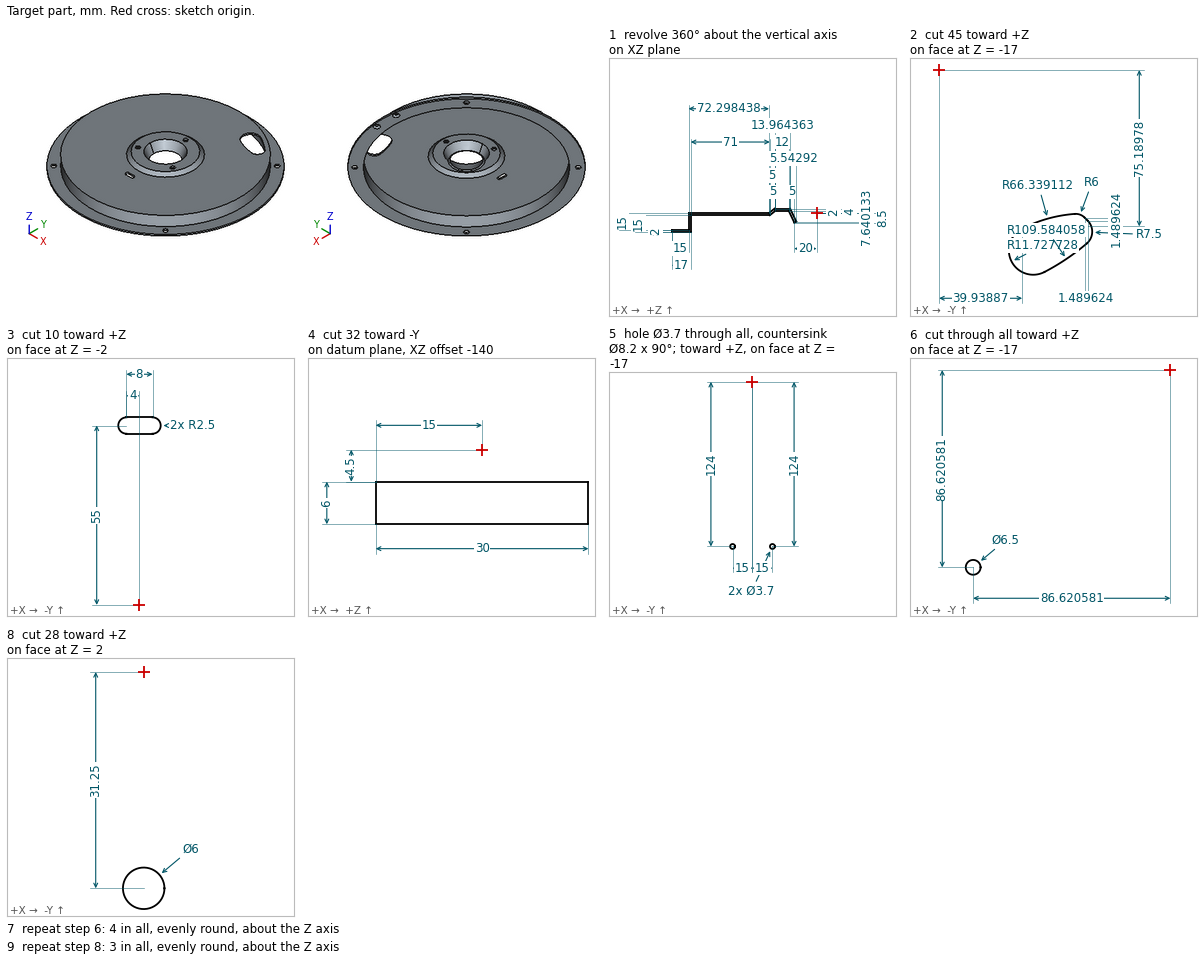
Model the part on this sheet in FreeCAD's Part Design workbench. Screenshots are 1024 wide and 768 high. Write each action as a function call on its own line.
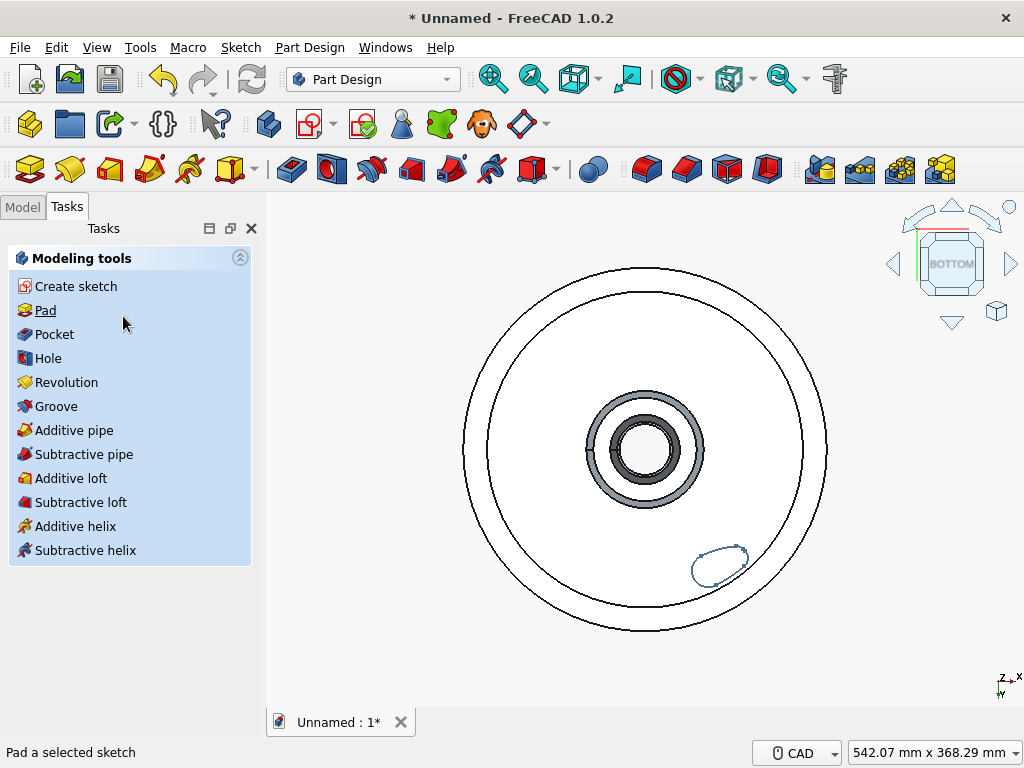
click(292, 170)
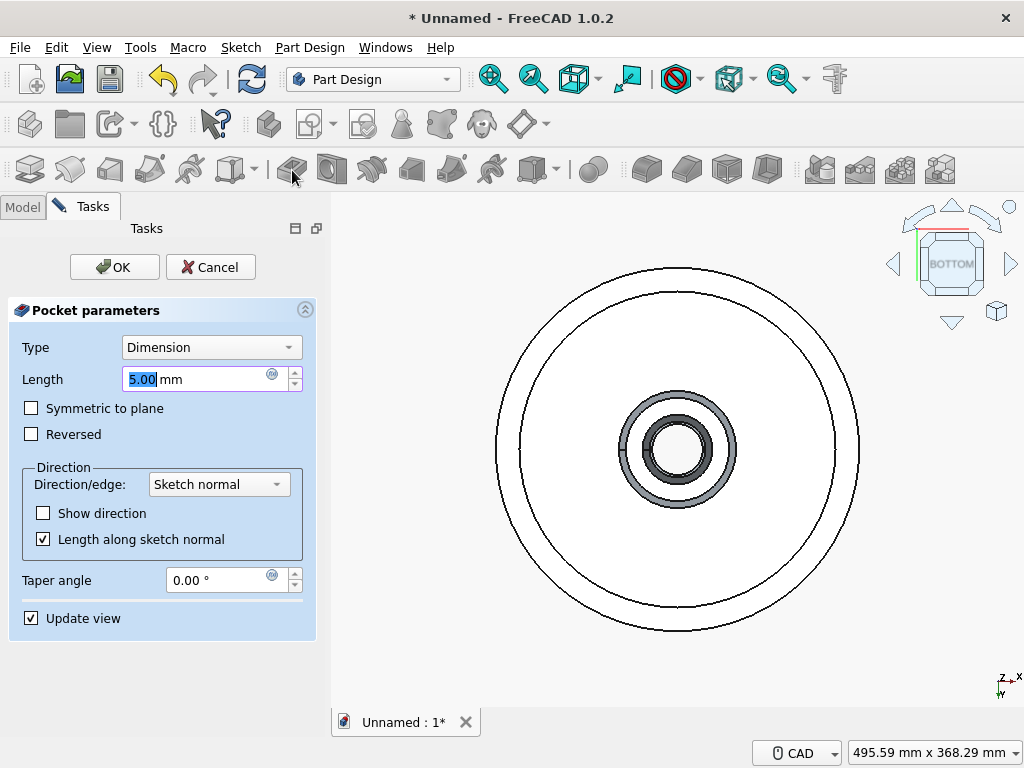
text(45)
key(Tab)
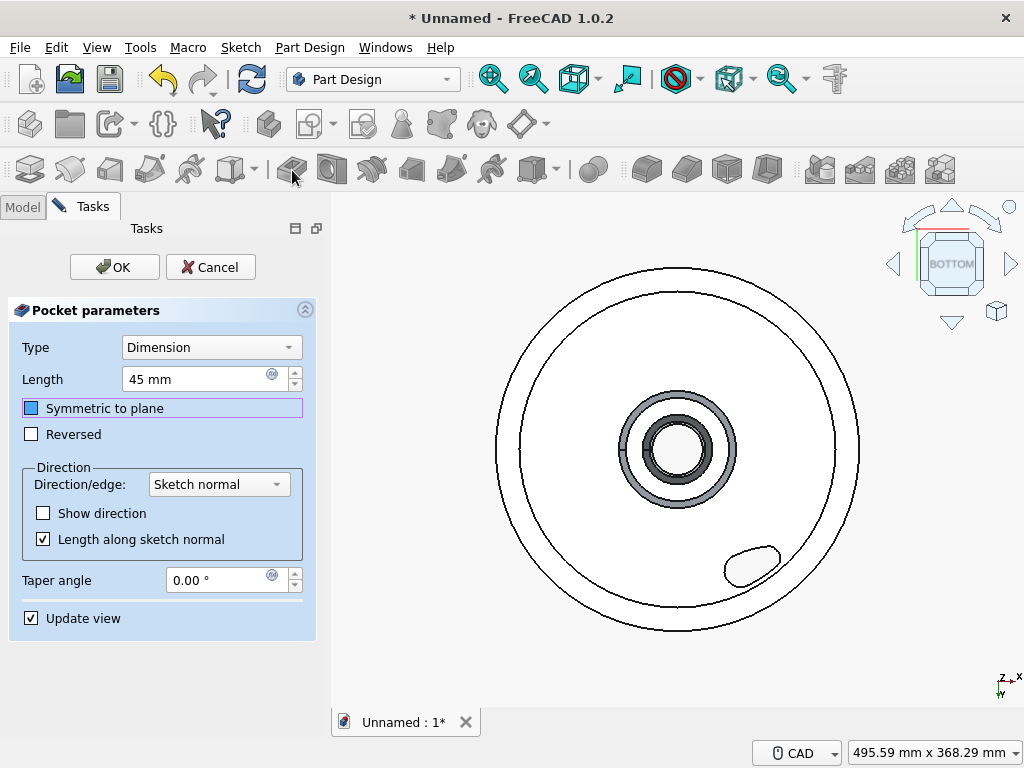
click(115, 267)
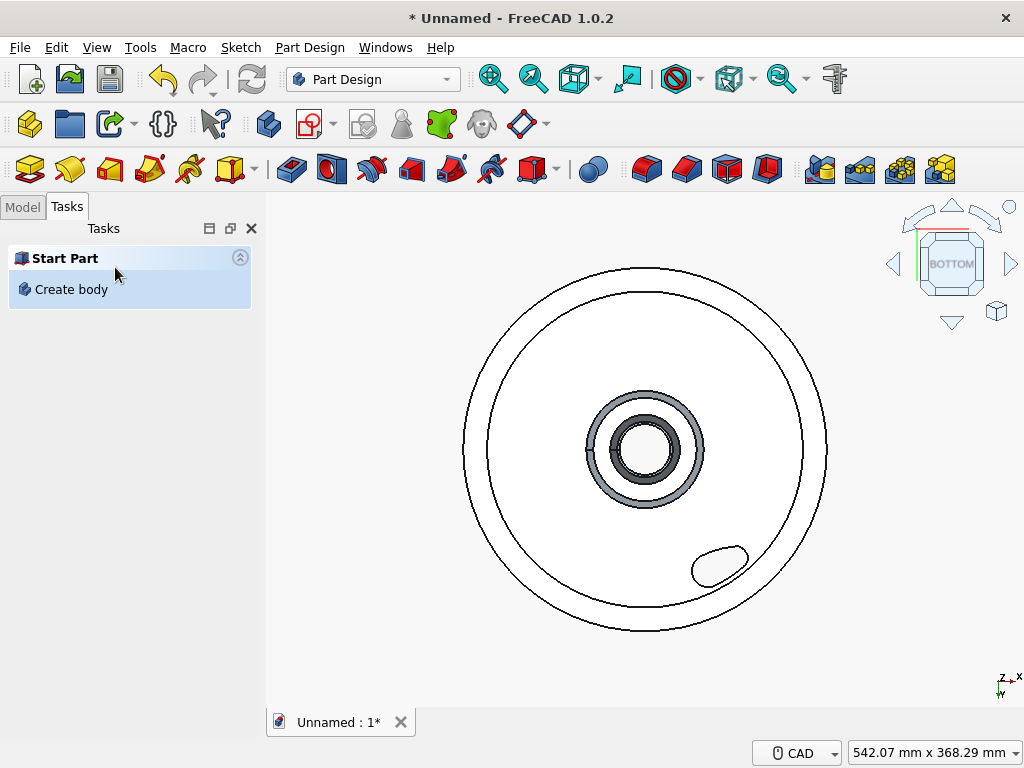
click(600, 358)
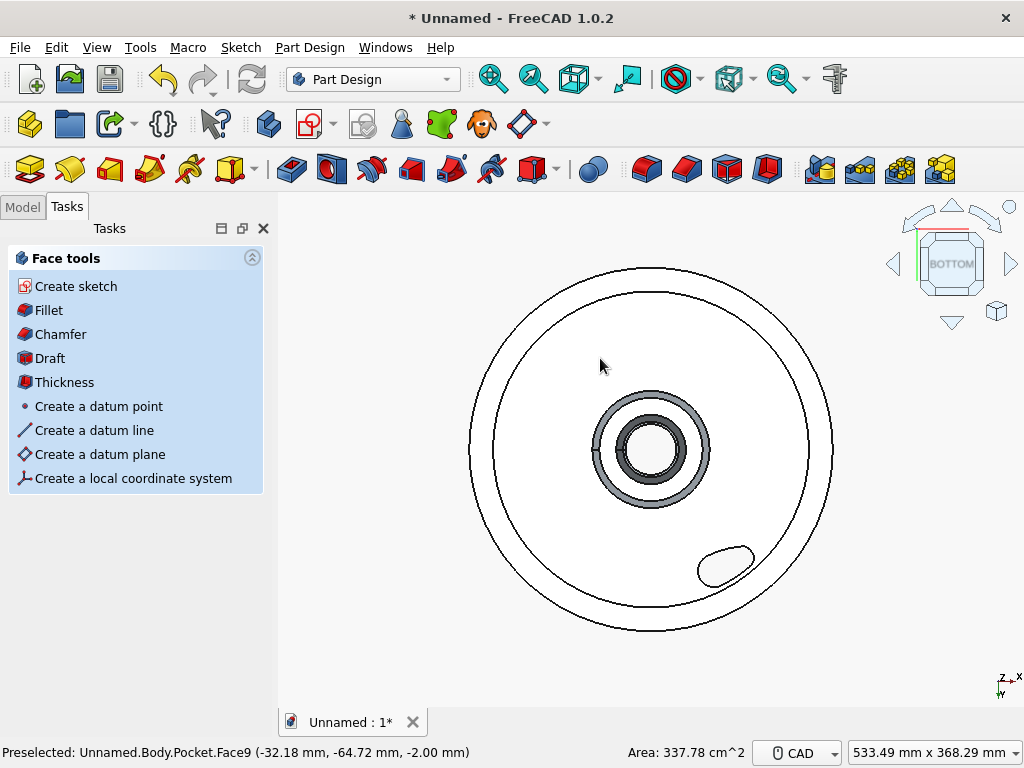
click(310, 124)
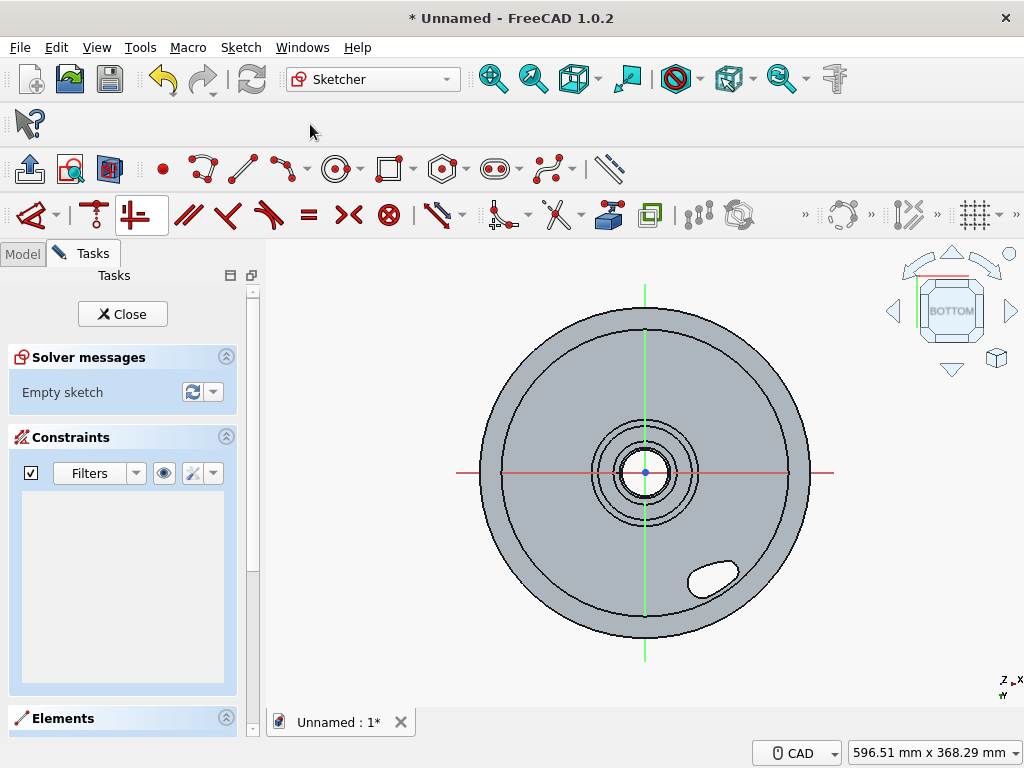
click(110, 170)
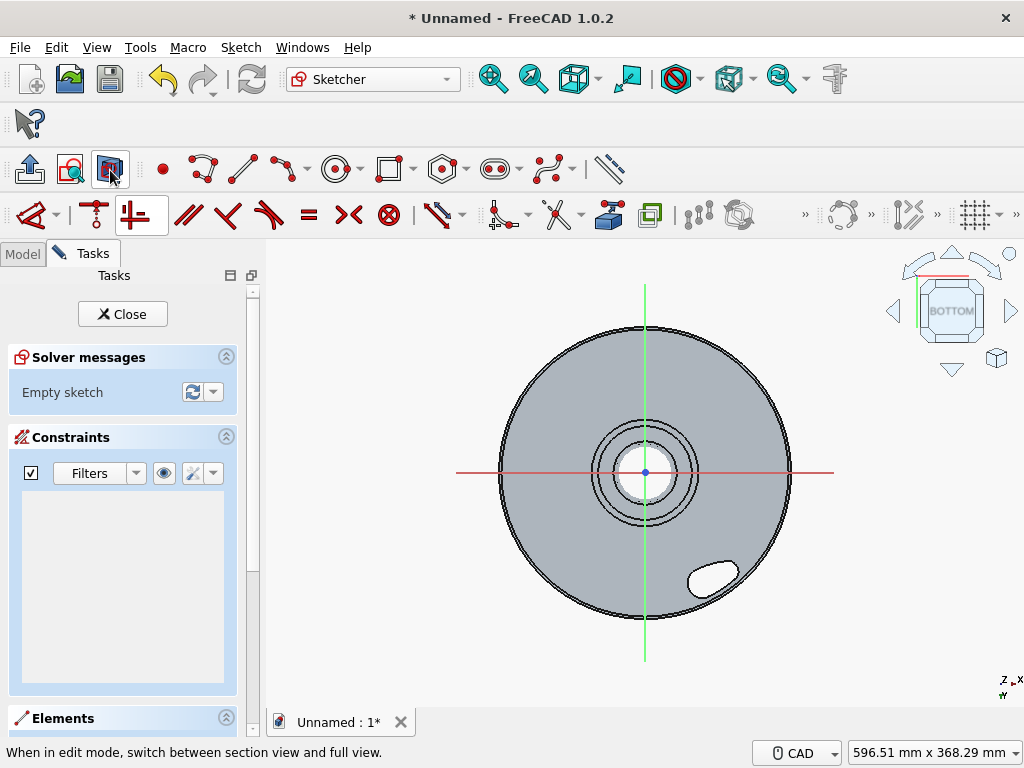
scroll(649, 399, up, 15)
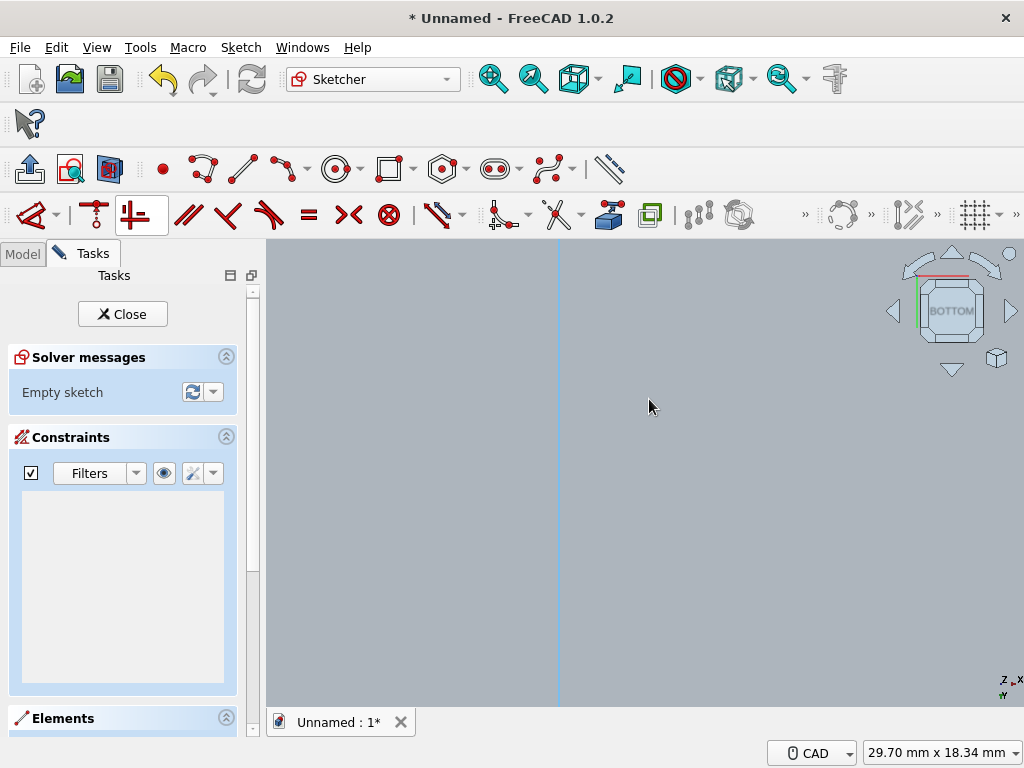
click(496, 170)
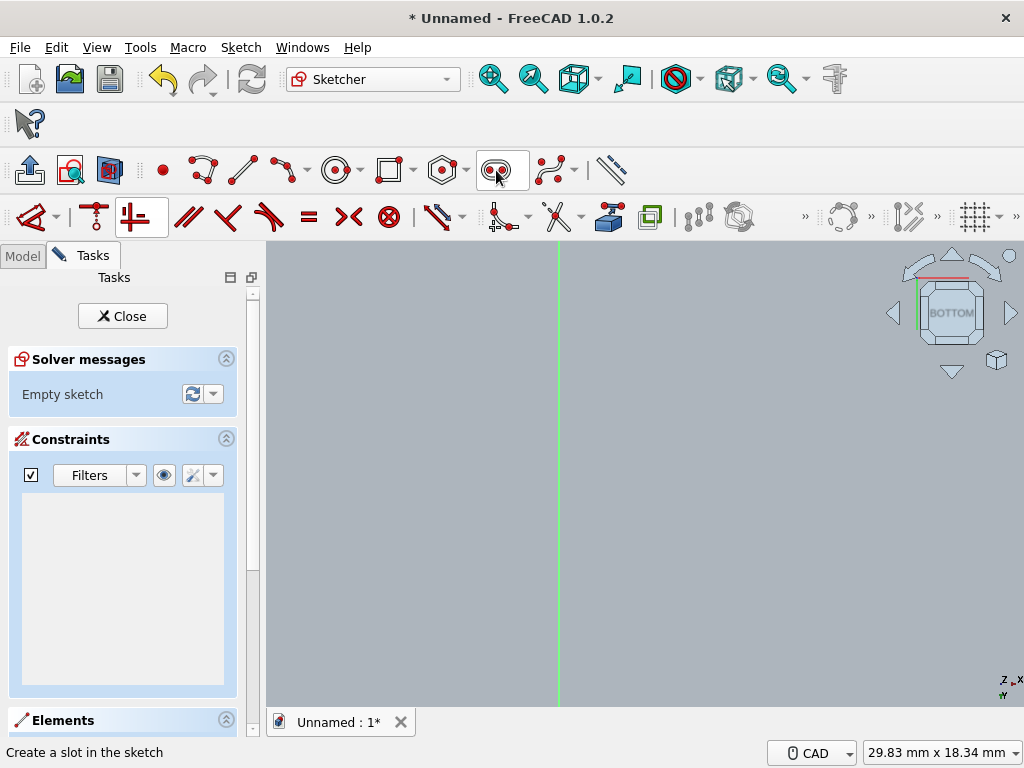
click(458, 476)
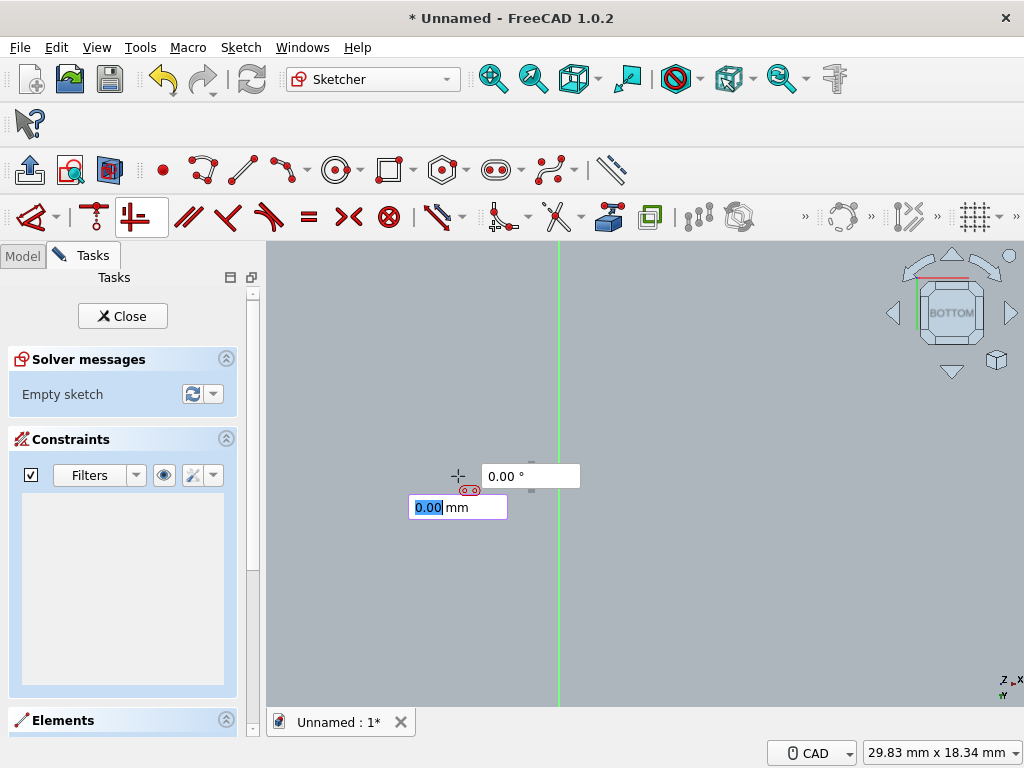
click(661, 476)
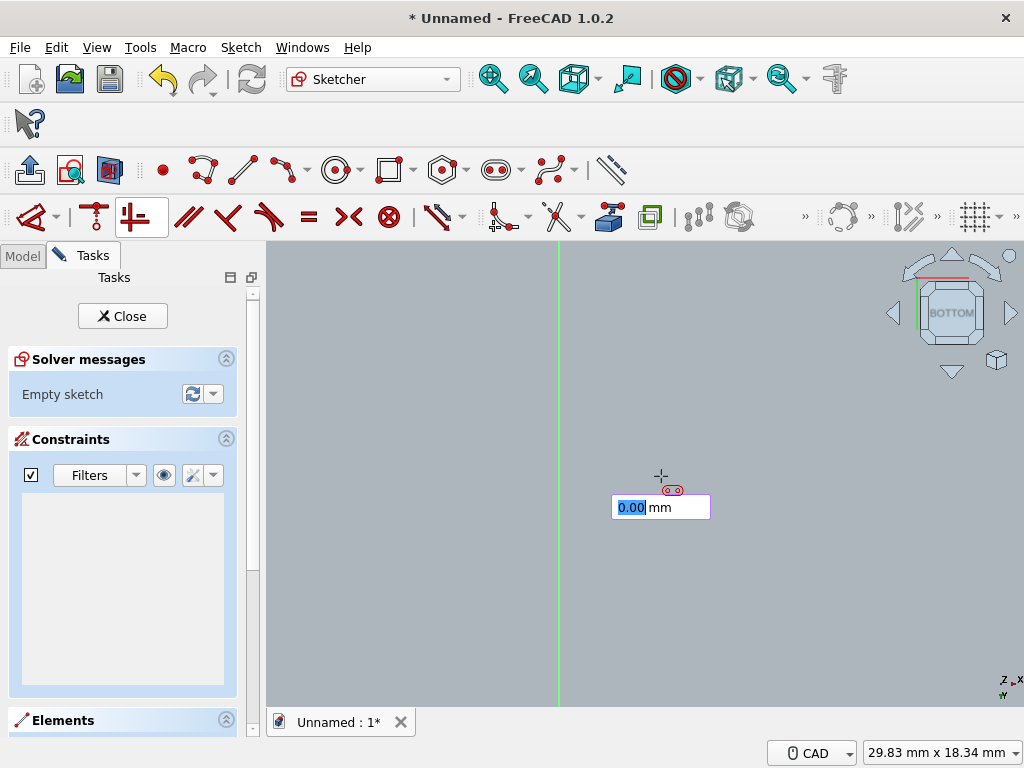
click(529, 540)
key(Escape)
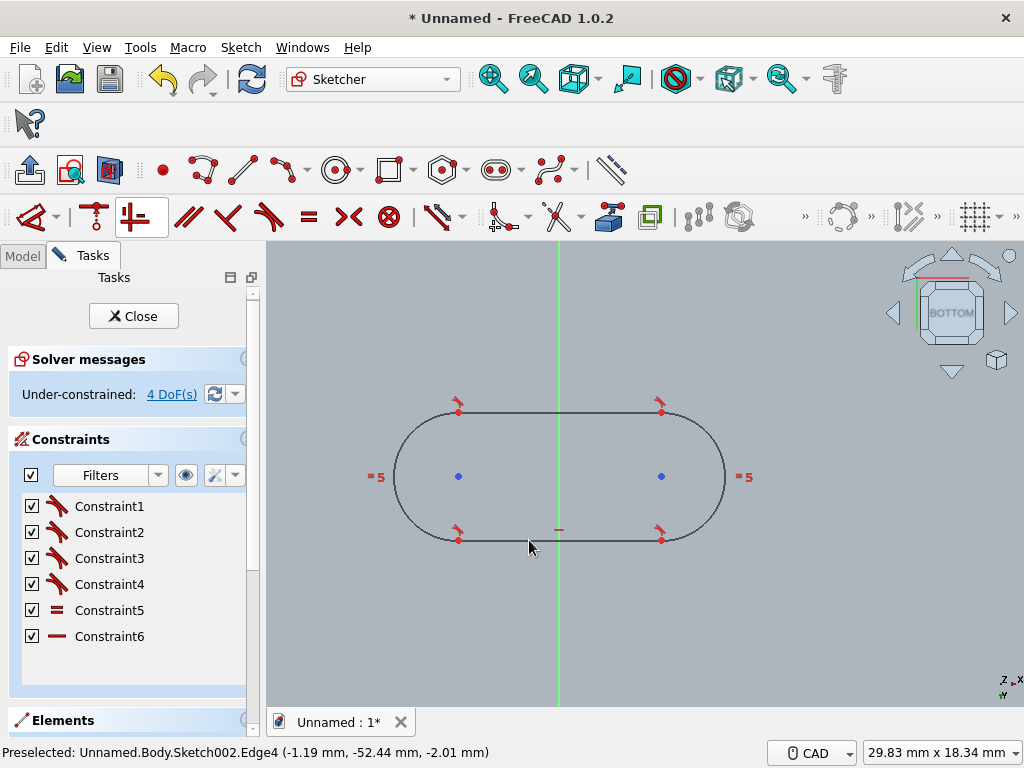
click(32, 218)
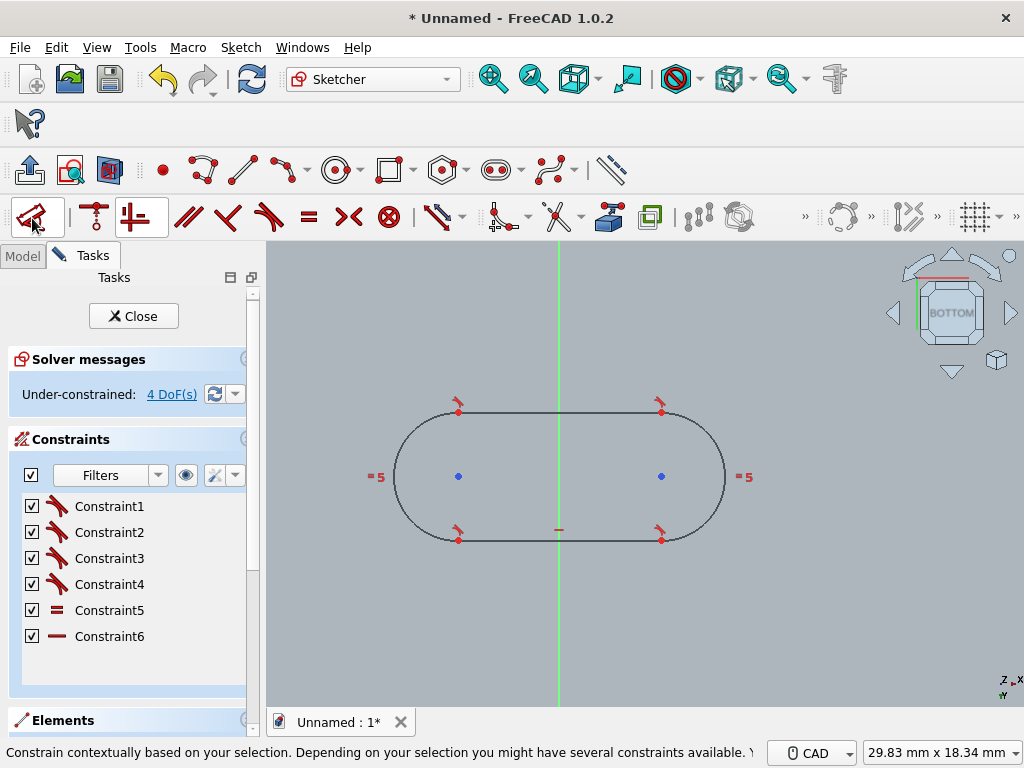
click(406, 439)
click(380, 420)